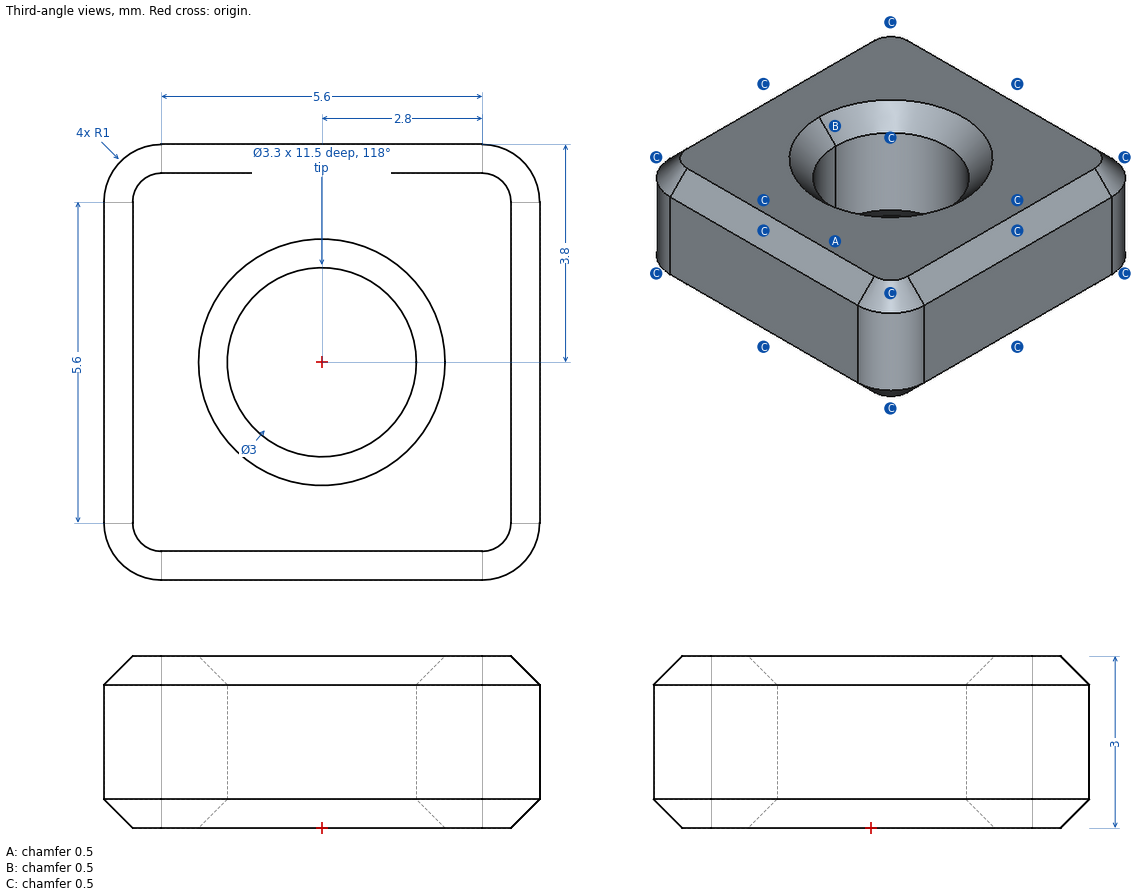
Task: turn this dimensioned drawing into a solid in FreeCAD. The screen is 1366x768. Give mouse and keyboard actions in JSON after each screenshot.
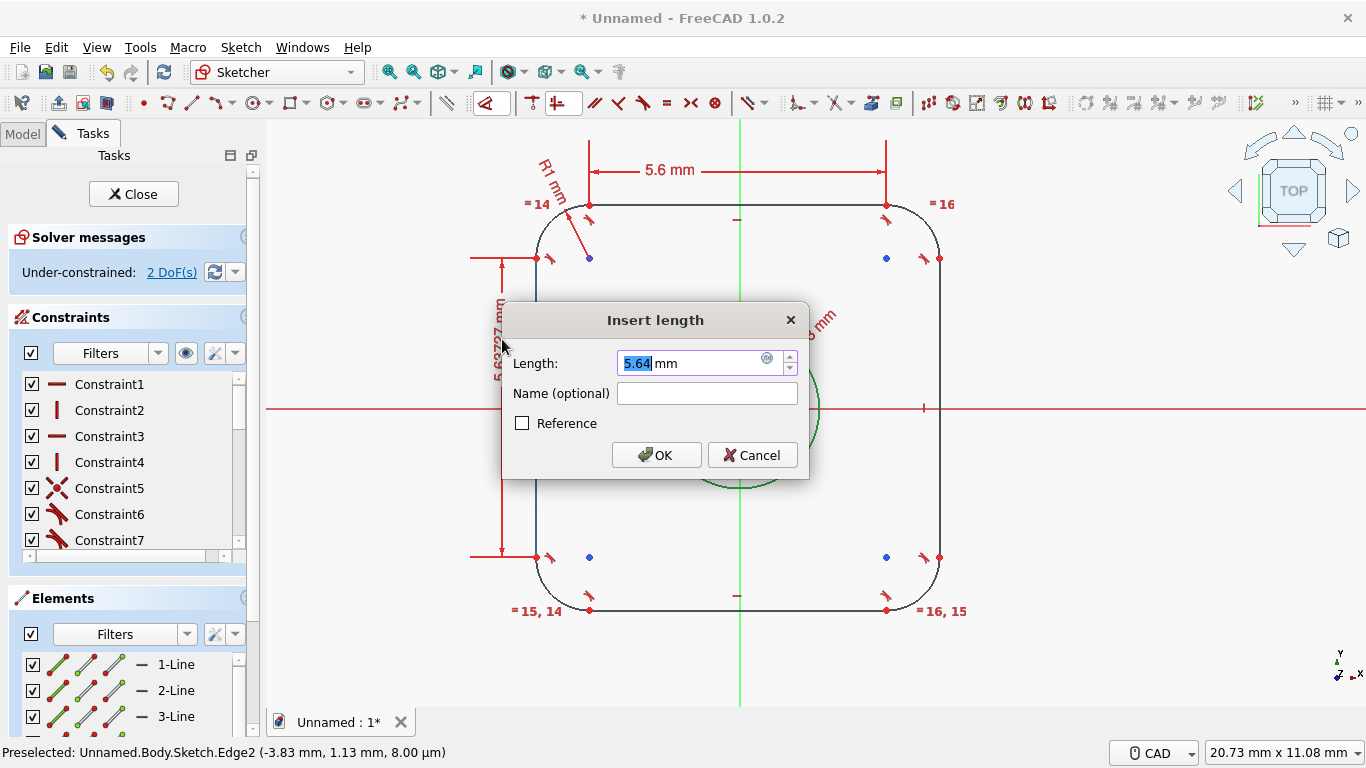
{"action": "type", "text": "5.6"}
{"action": "key", "text": "Return"}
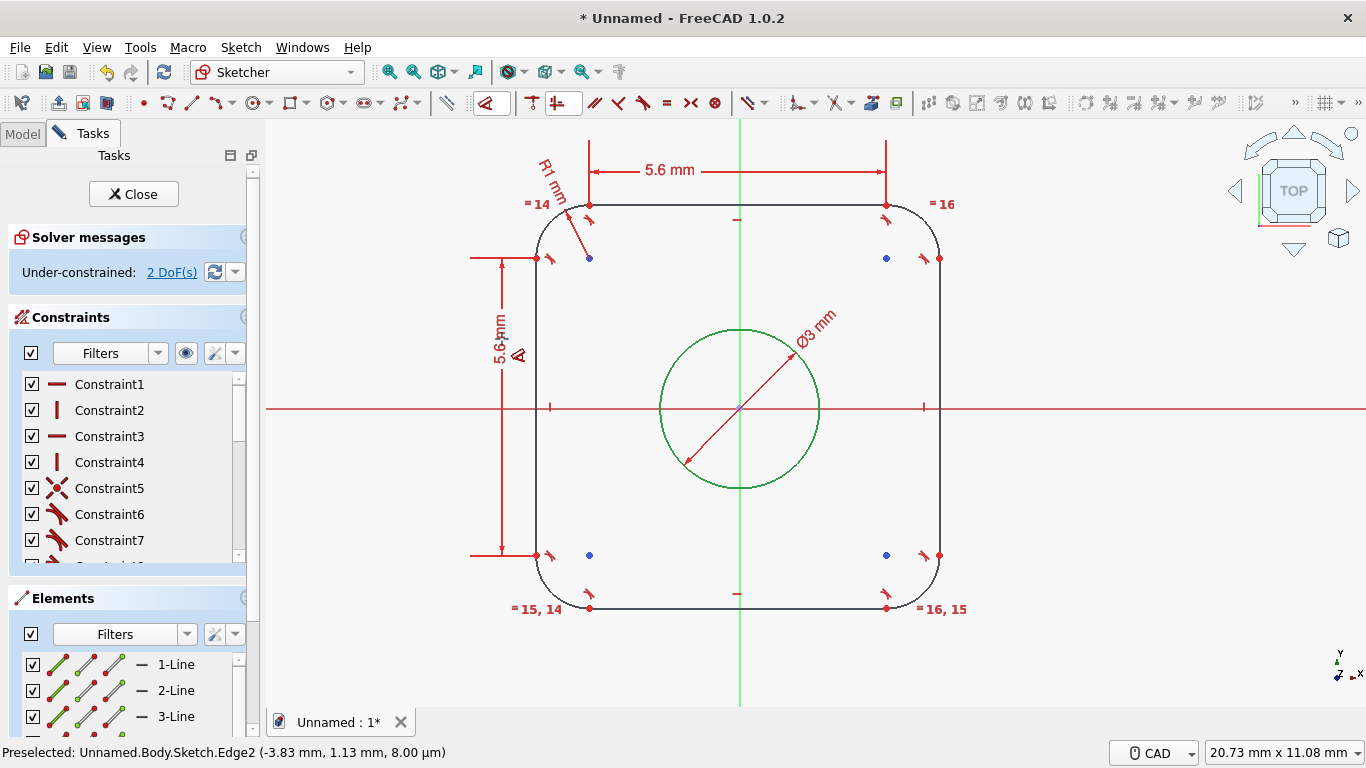
{"action": "left_click", "coordinate": [886, 205]}
{"action": "left_click", "coordinate": [813, 171]}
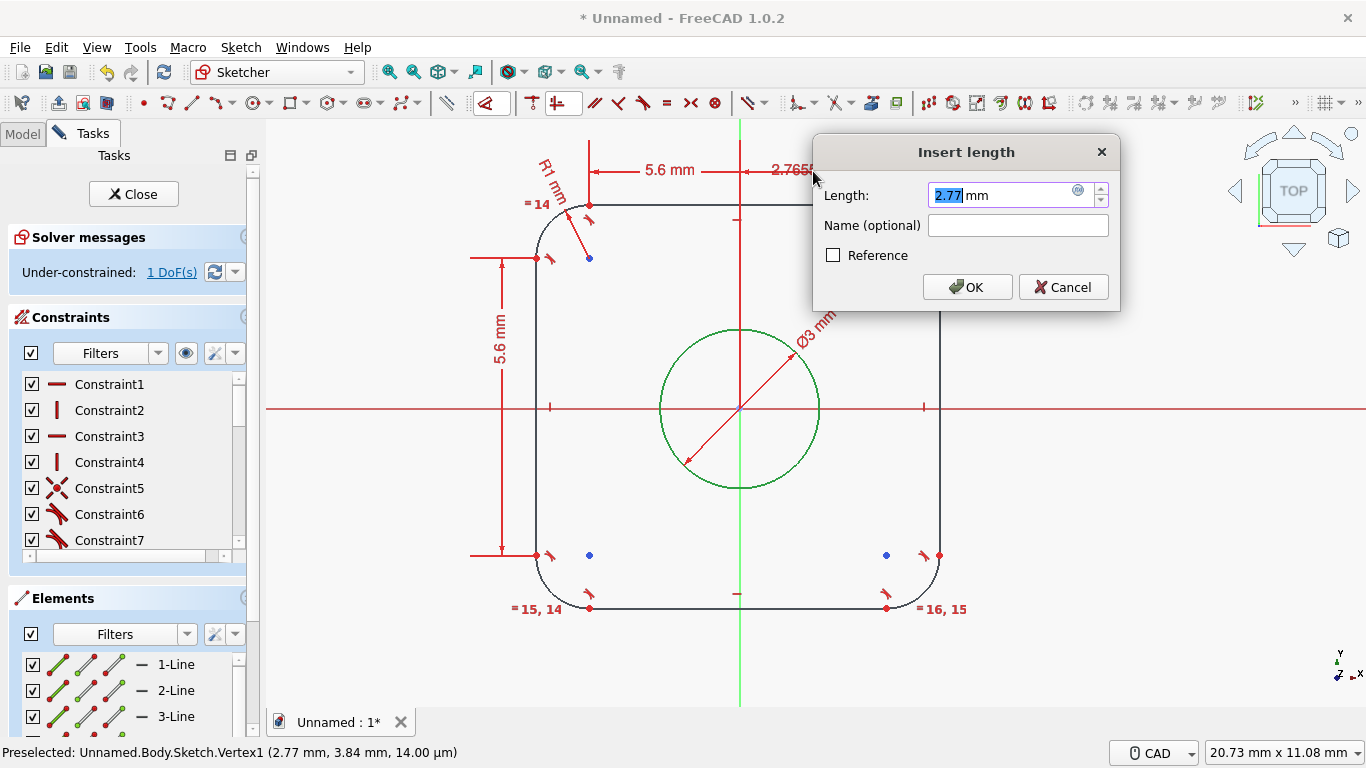
{"action": "type", "text": "2.8"}
{"action": "key", "text": "Return"}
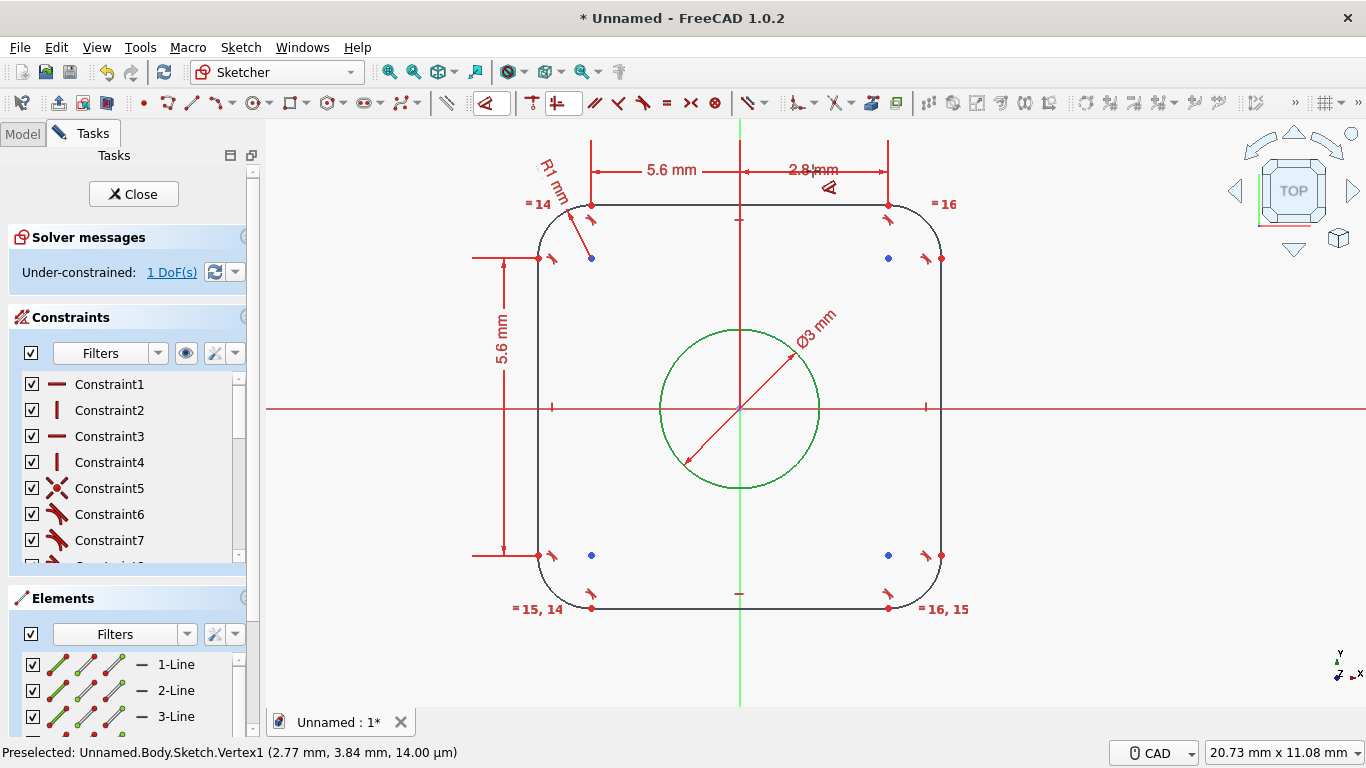
{"action": "left_click", "coordinate": [888, 205]}
{"action": "left_click", "coordinate": [922, 307]}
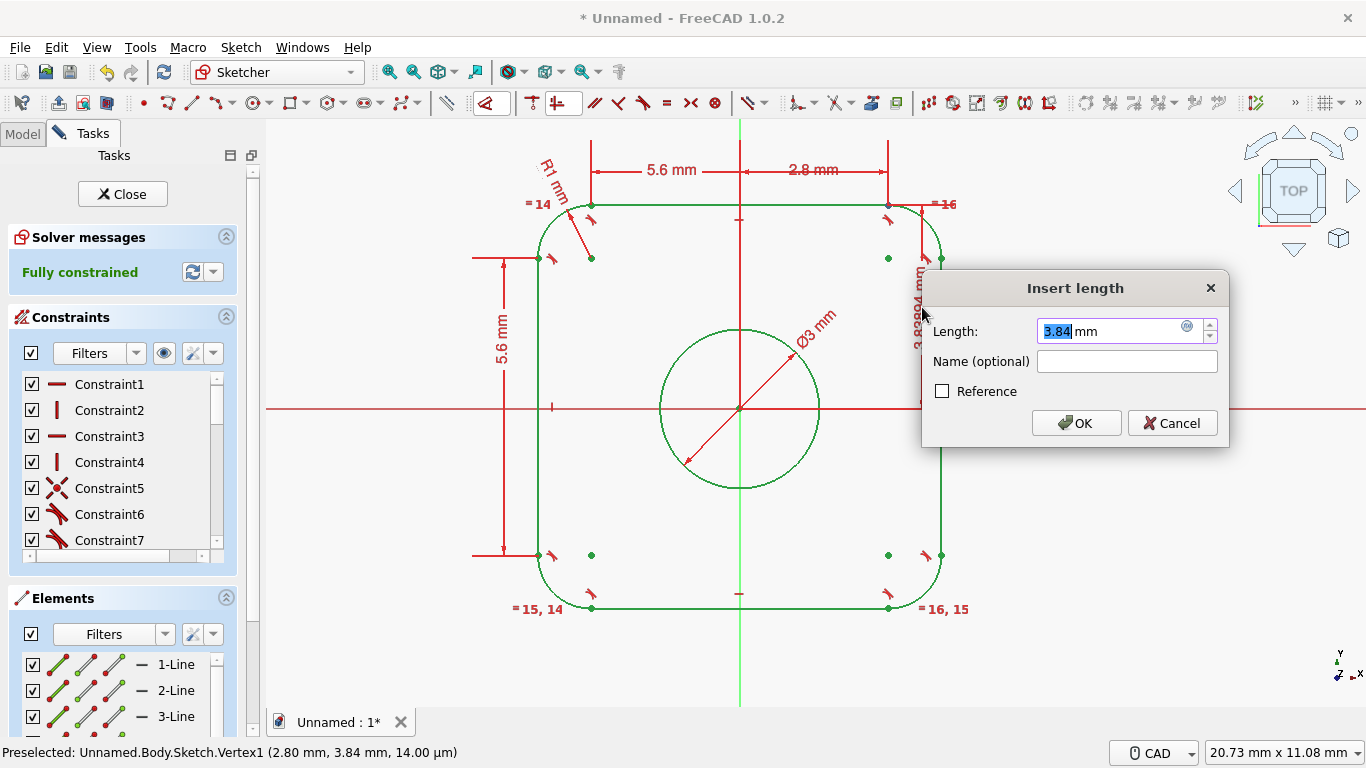
{"action": "type", "text": "3.8"}
{"action": "key", "text": "Return"}
{"action": "key", "text": "Escape"}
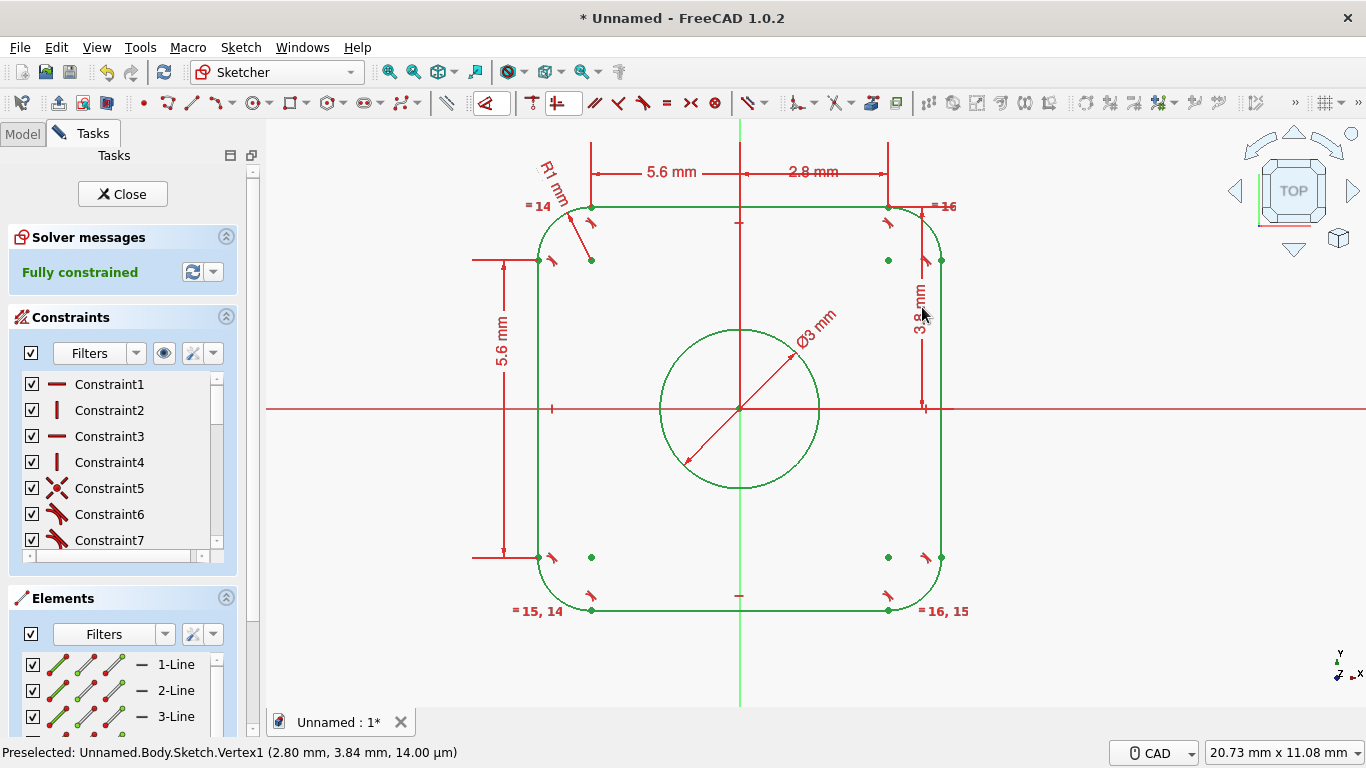
{"action": "left_click", "coordinate": [123, 194]}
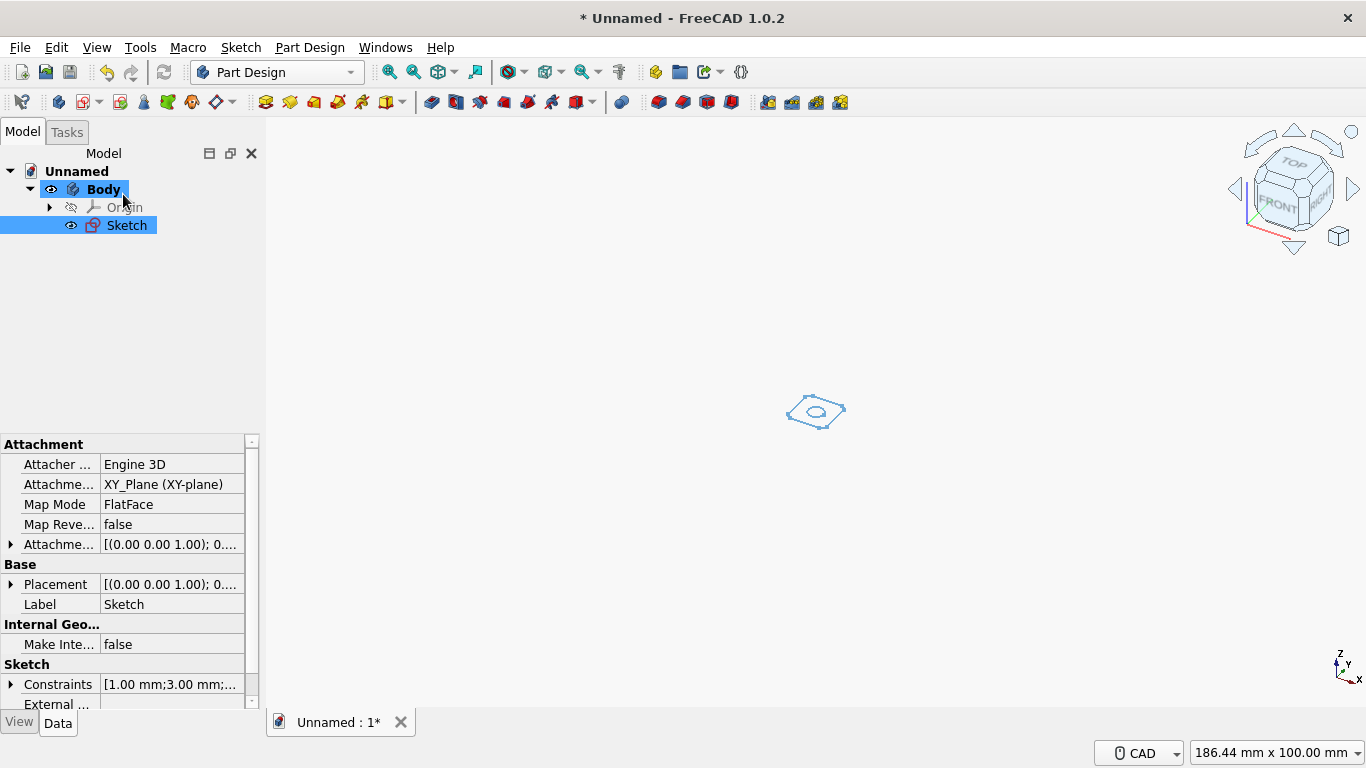
{"action": "left_click", "coordinate": [266, 102]}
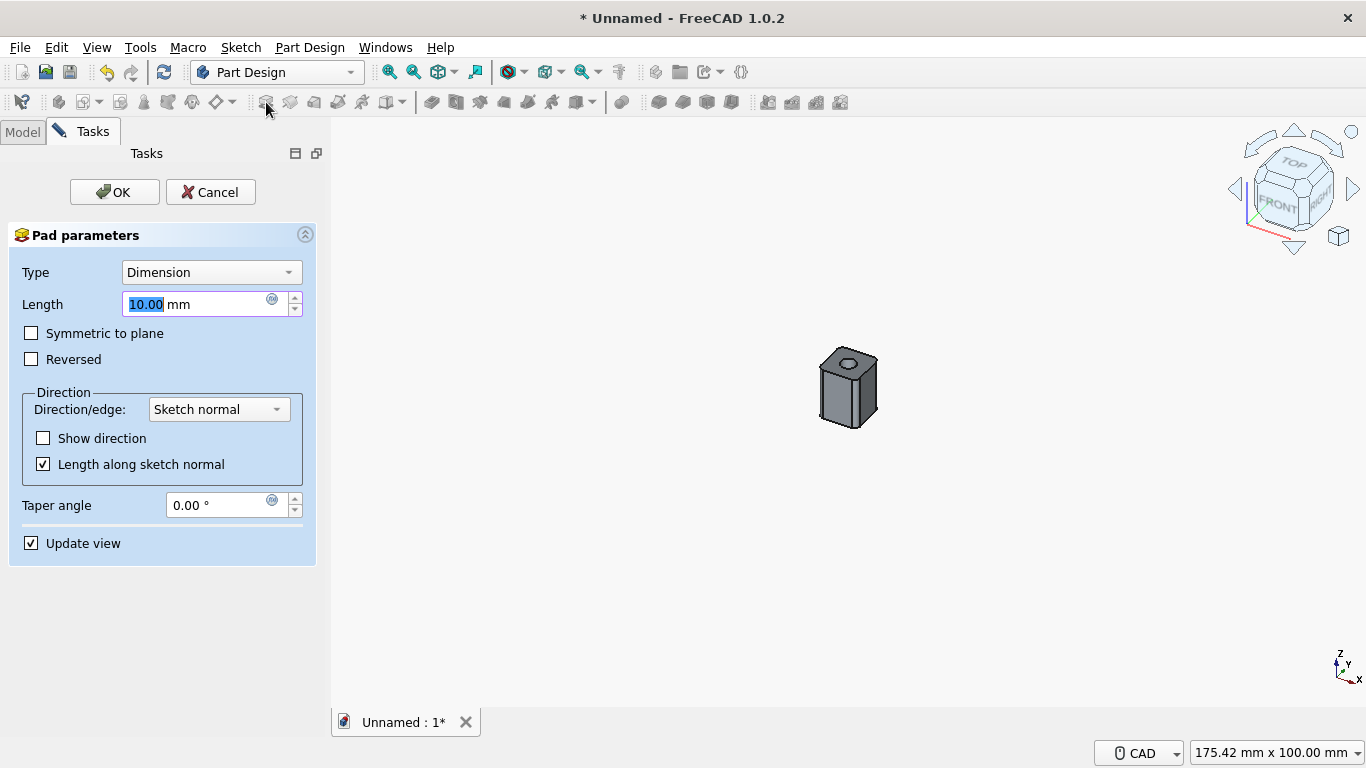
{"action": "type", "text": "3"}
{"action": "key", "text": "Tab"}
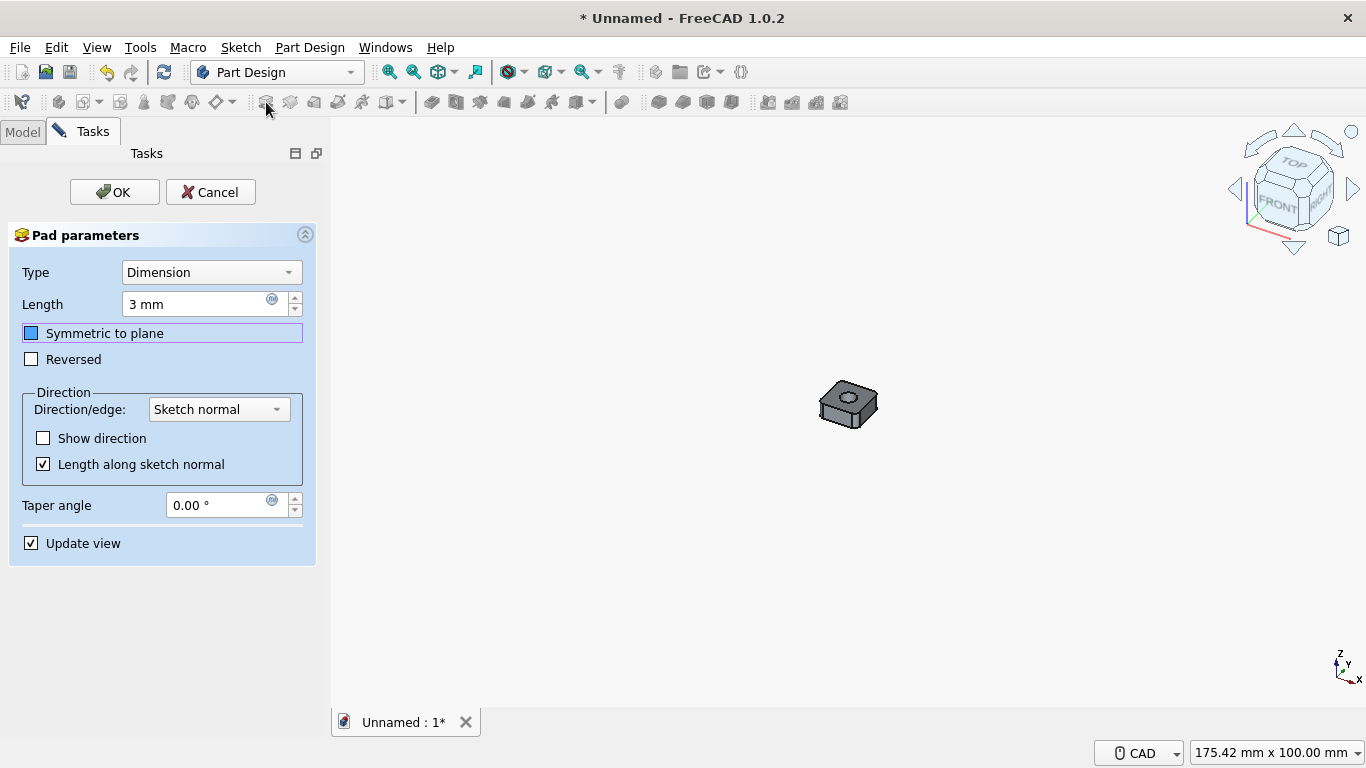
{"action": "left_click", "coordinate": [115, 192]}